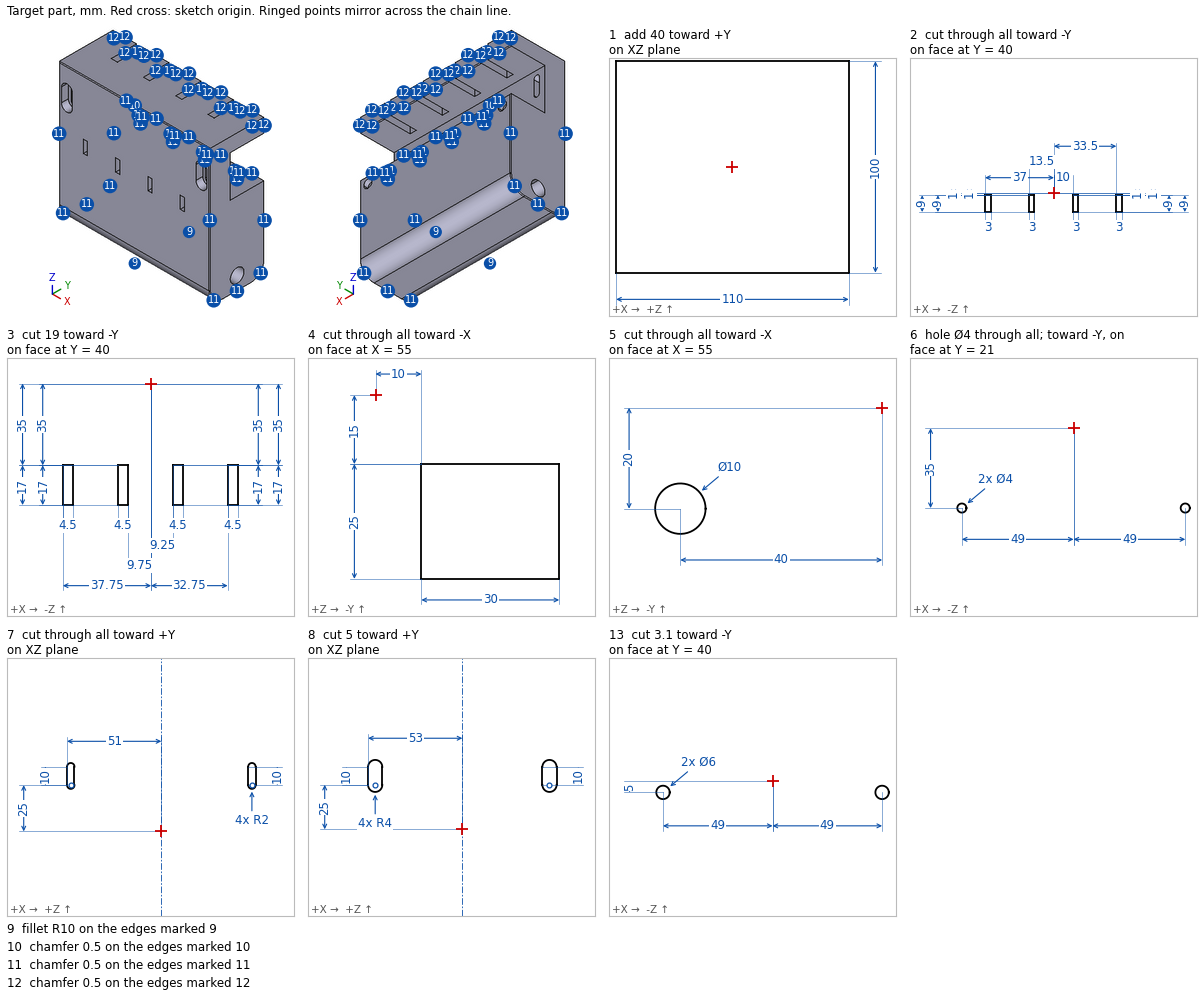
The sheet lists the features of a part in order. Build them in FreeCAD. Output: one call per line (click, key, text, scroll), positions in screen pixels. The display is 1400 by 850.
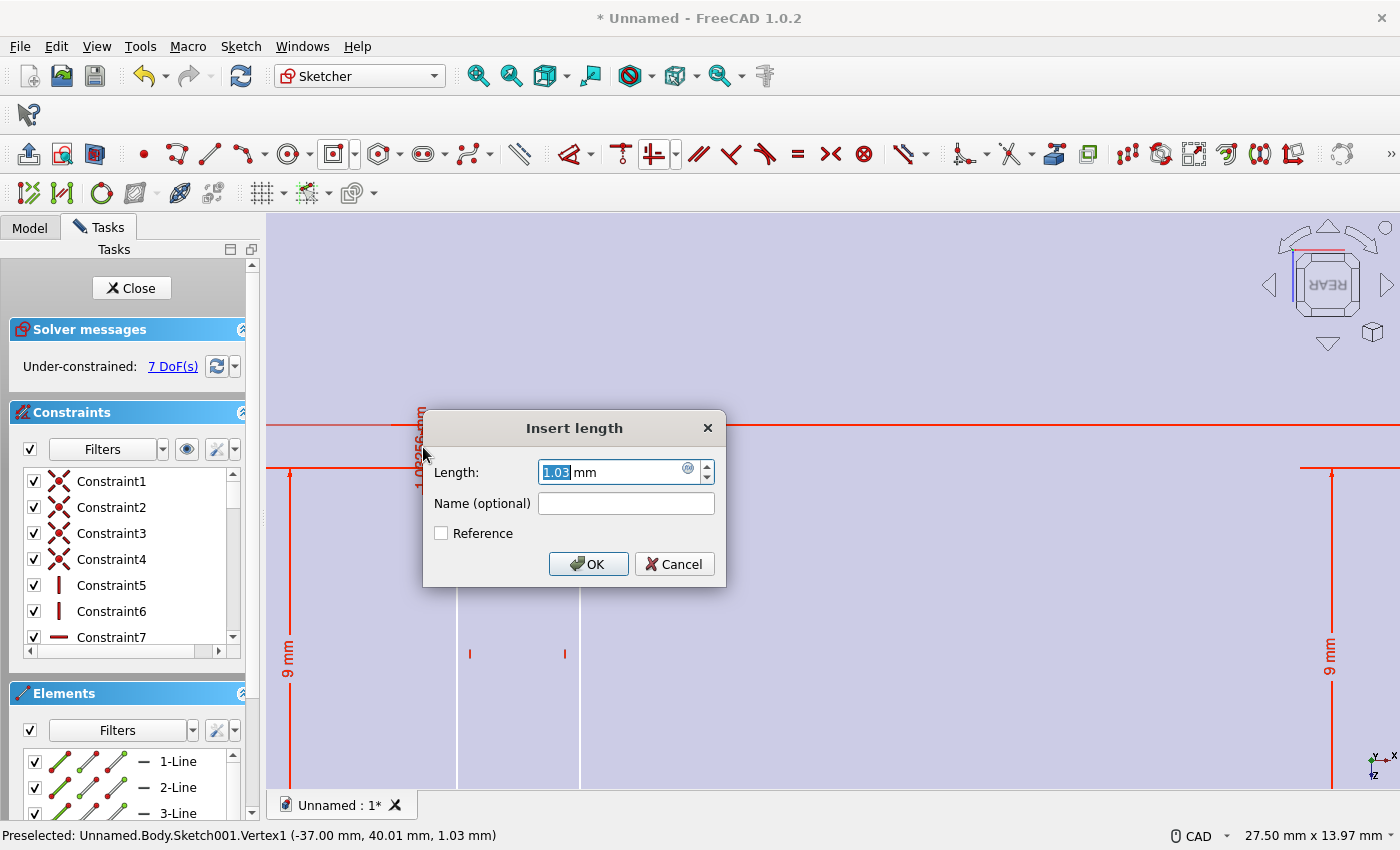
text(1)
key(Return)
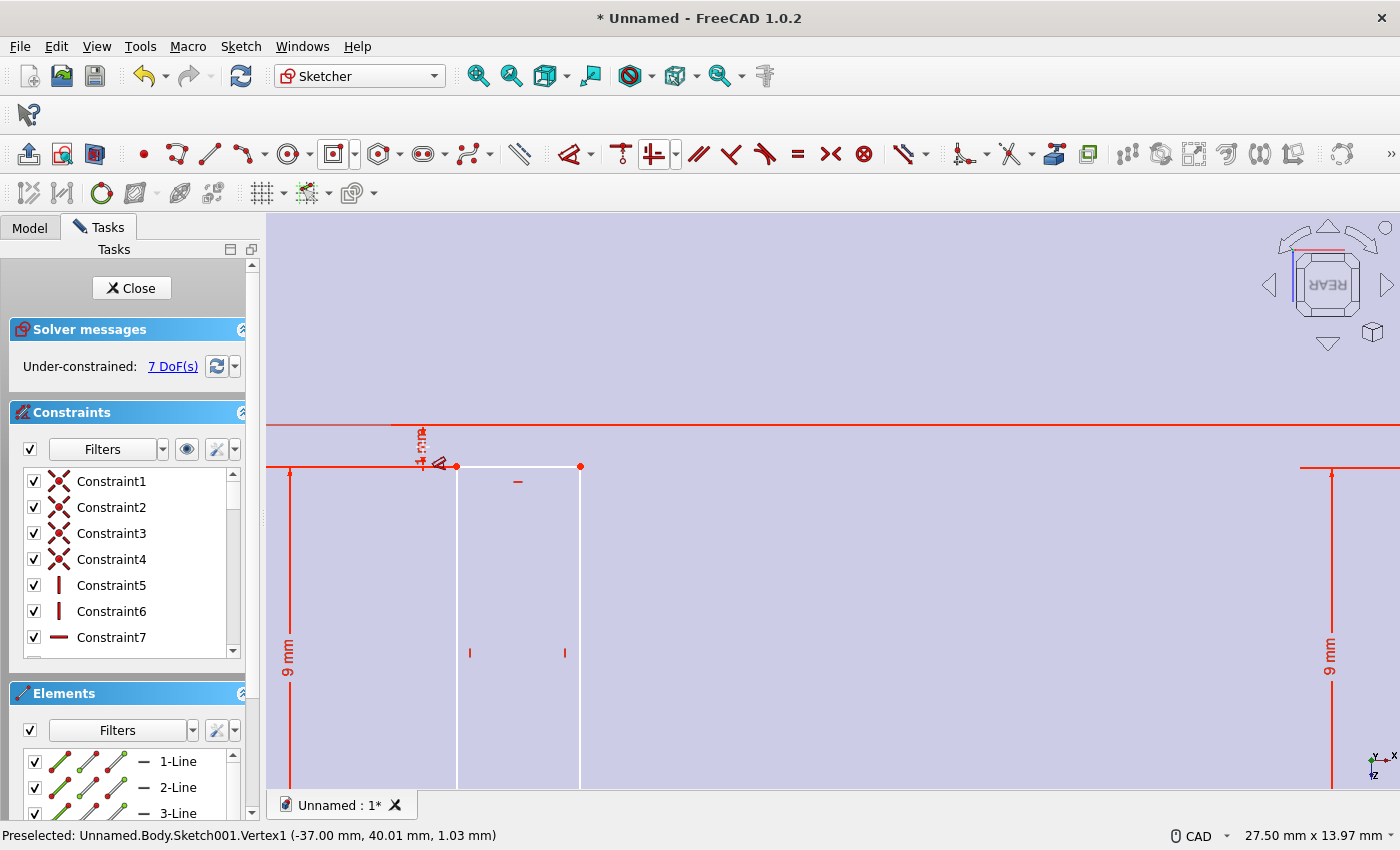
scroll(459, 468, down, 8)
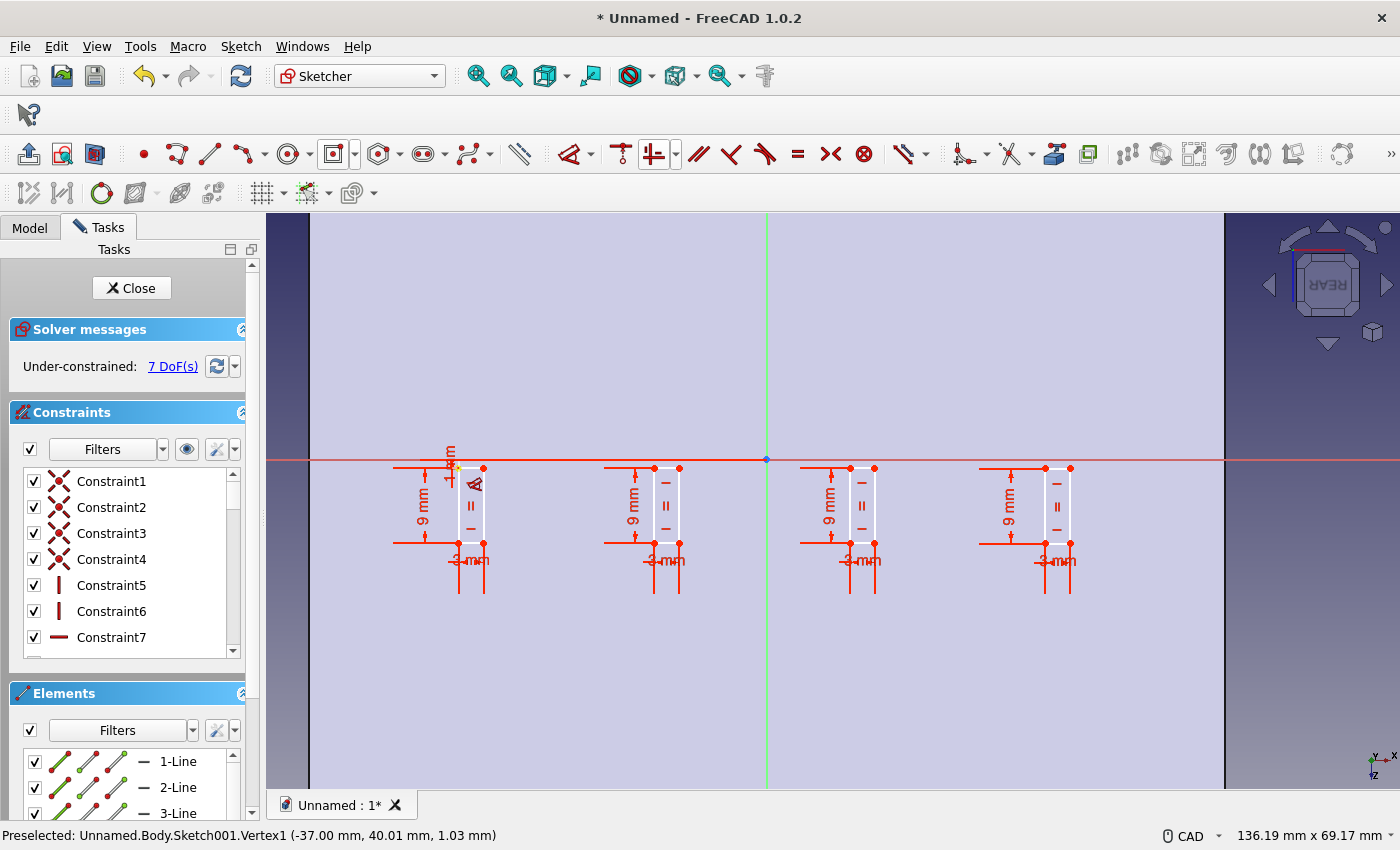
scroll(654, 468, up, 8)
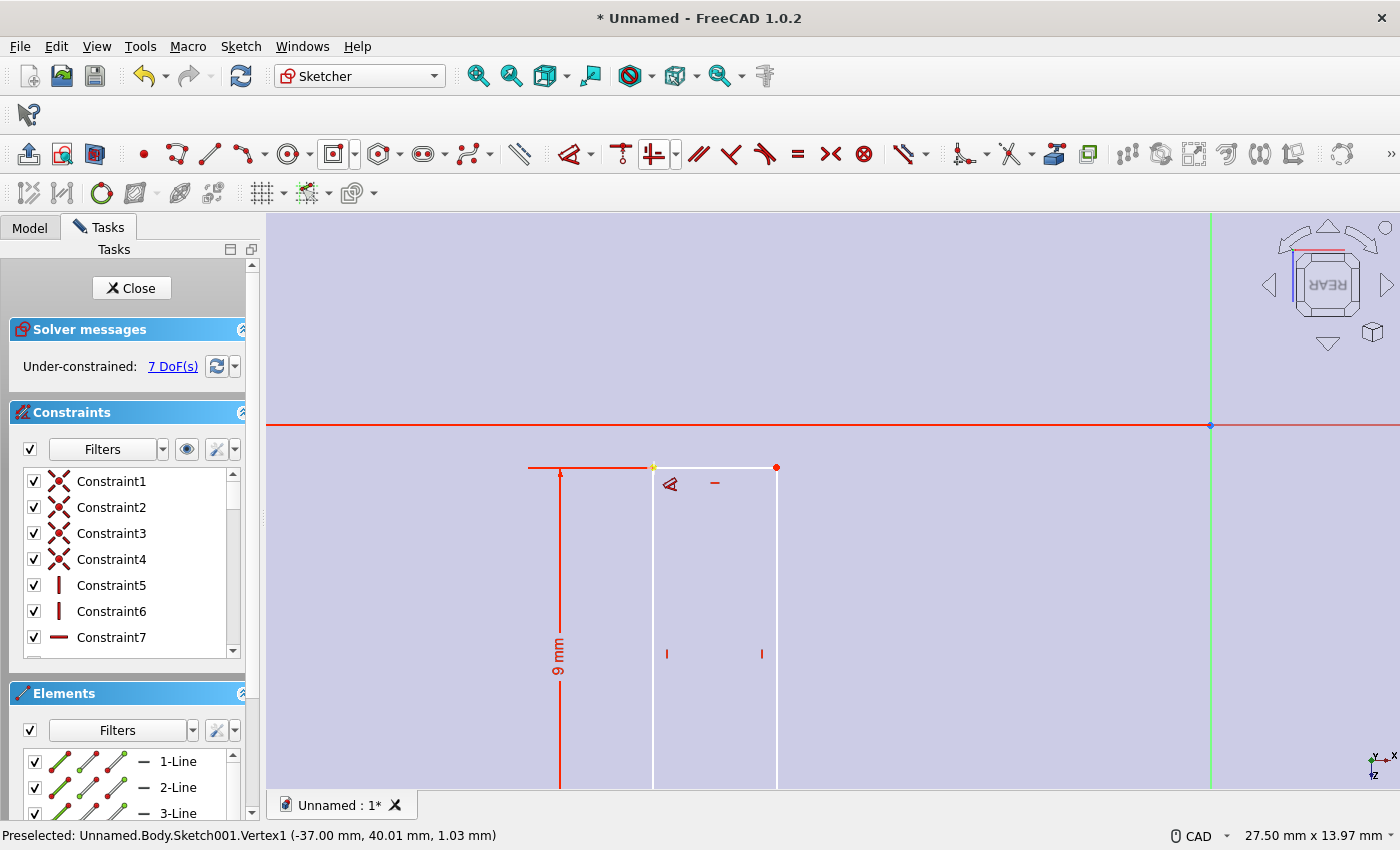
click(653, 468)
click(619, 447)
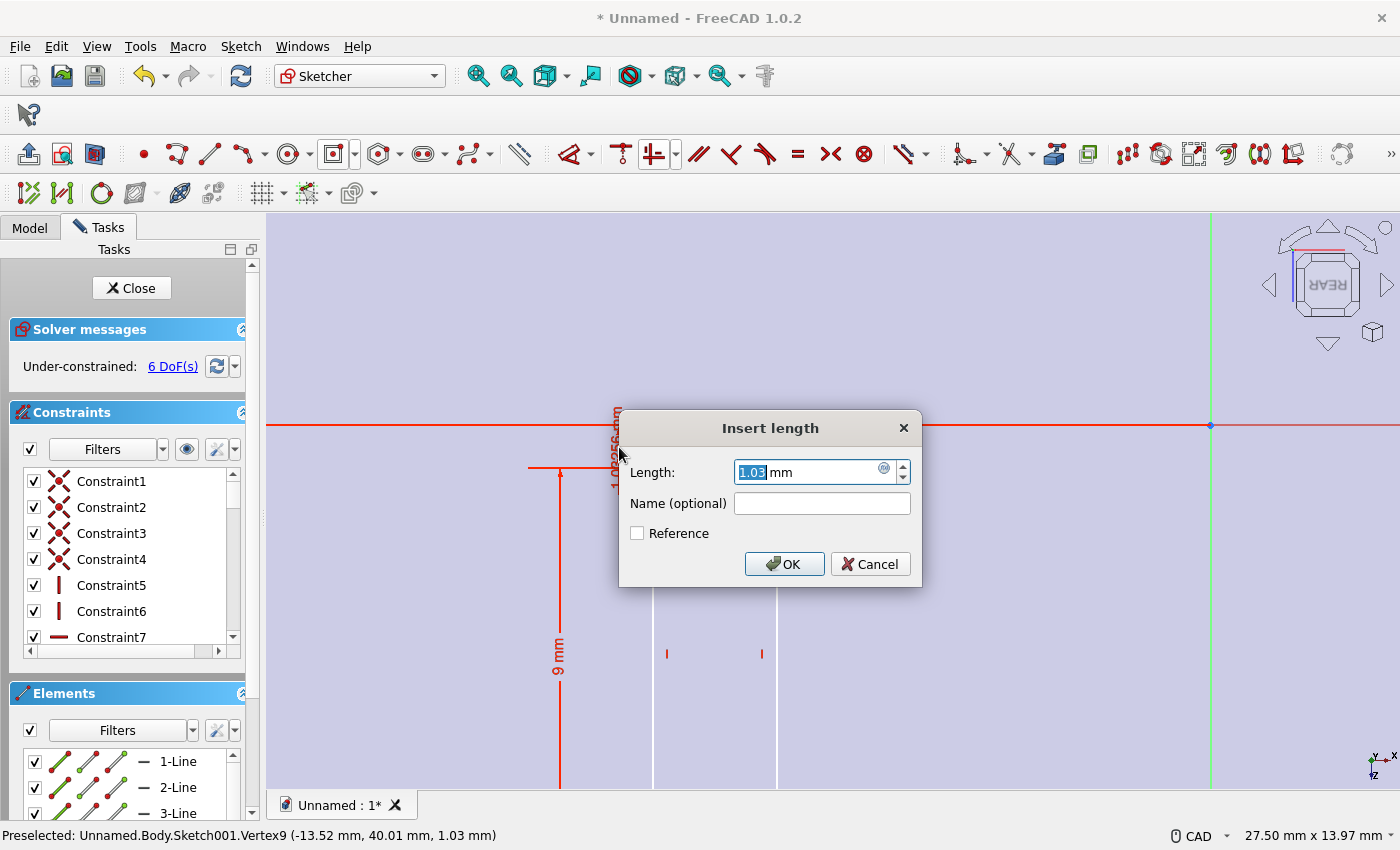
text(1)
key(Return)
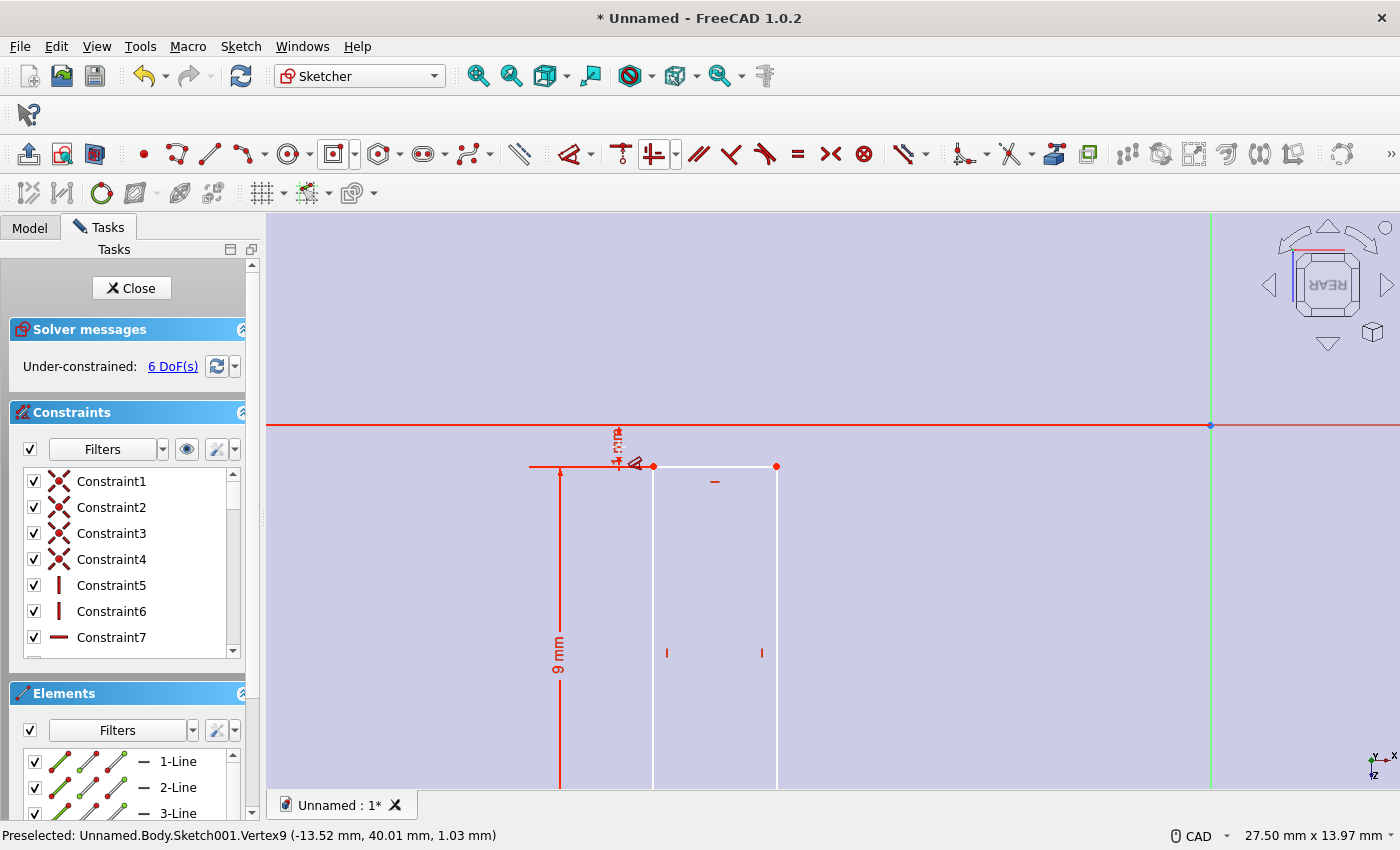
scroll(654, 468, down, 8)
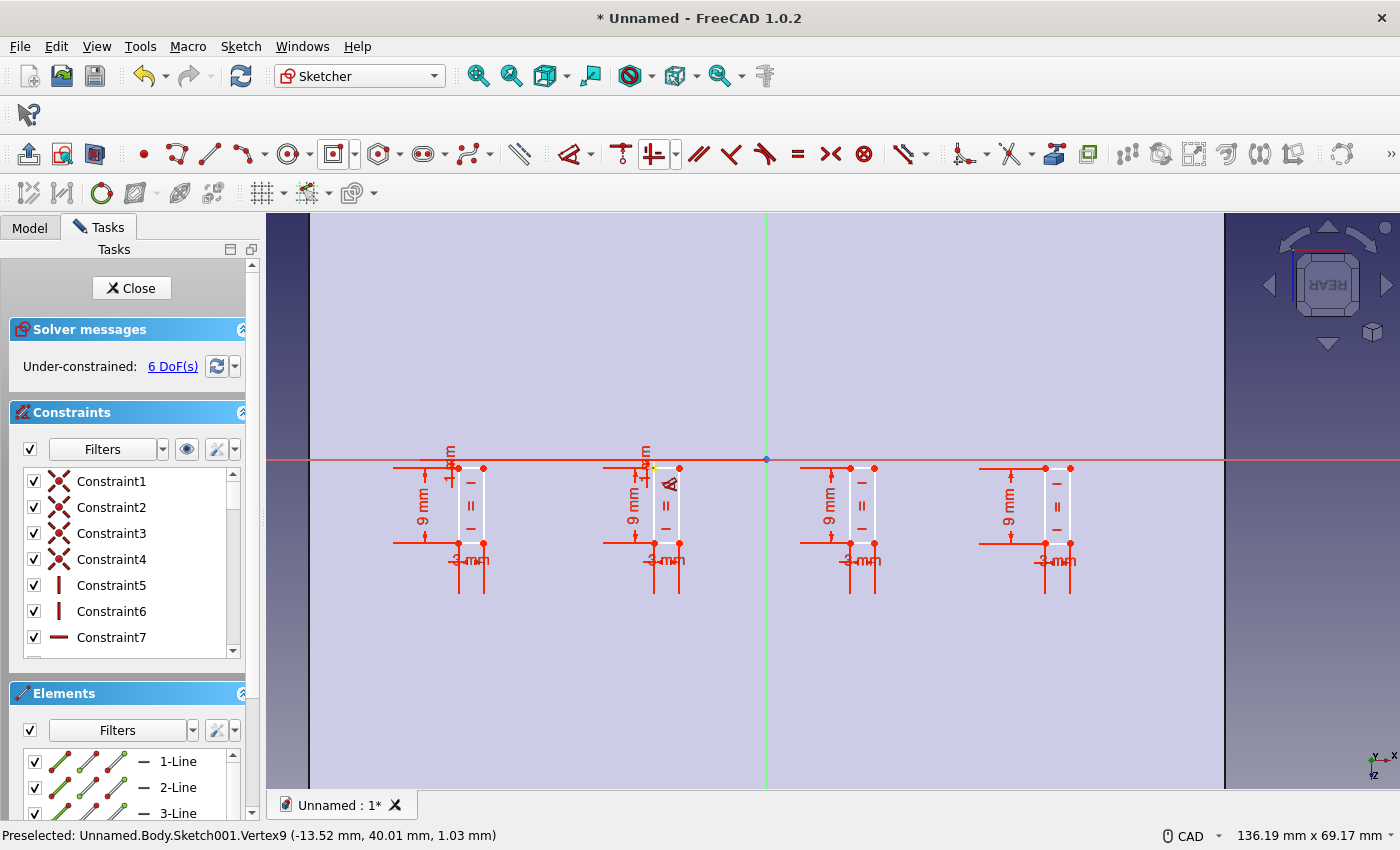
scroll(850, 468, up, 8)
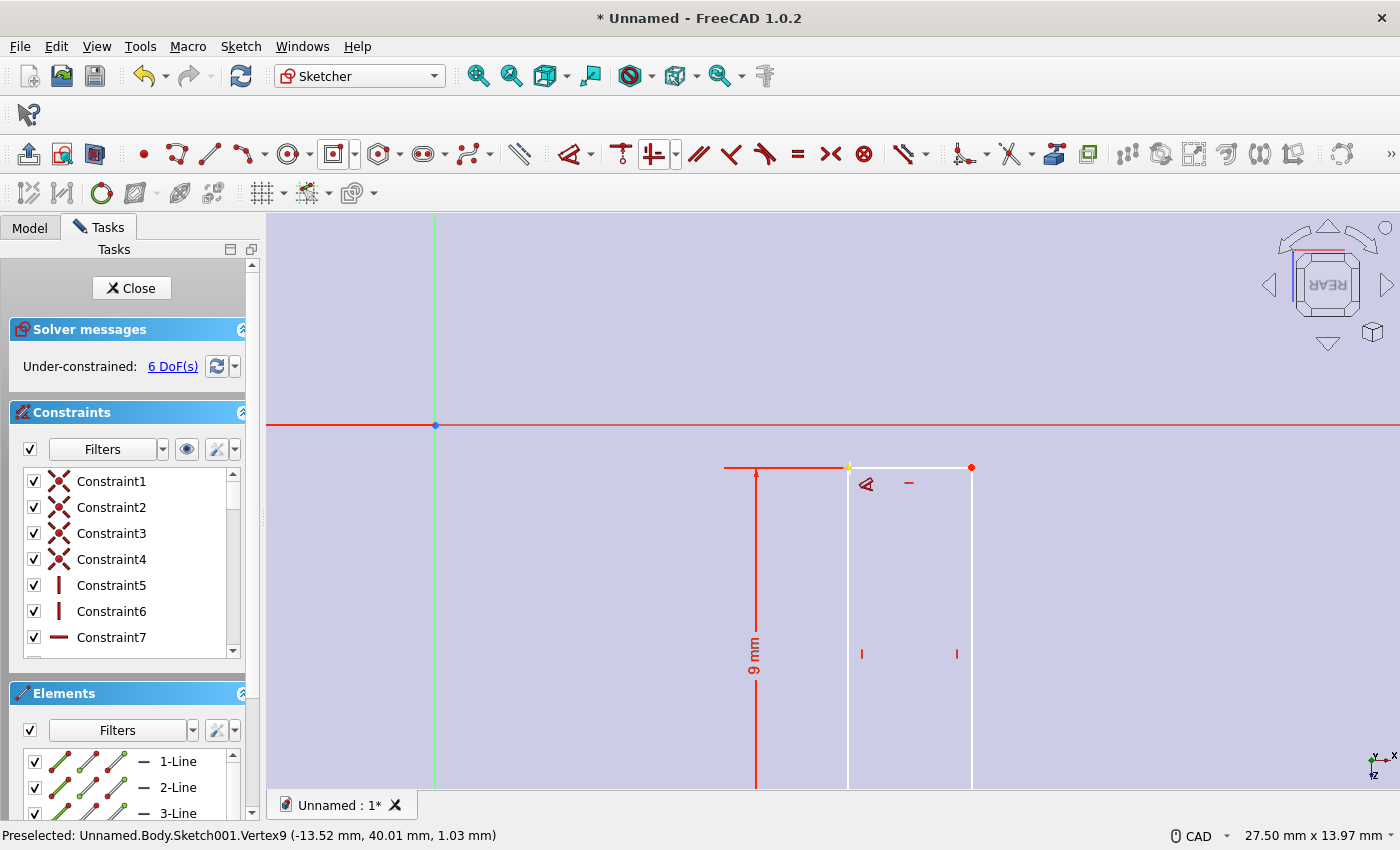
click(848, 468)
click(882, 447)